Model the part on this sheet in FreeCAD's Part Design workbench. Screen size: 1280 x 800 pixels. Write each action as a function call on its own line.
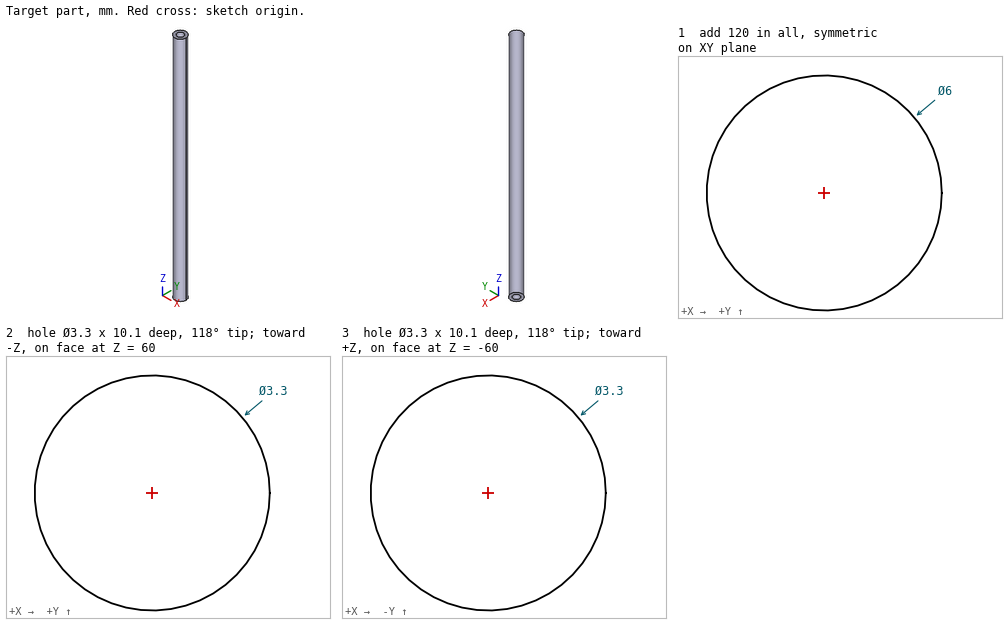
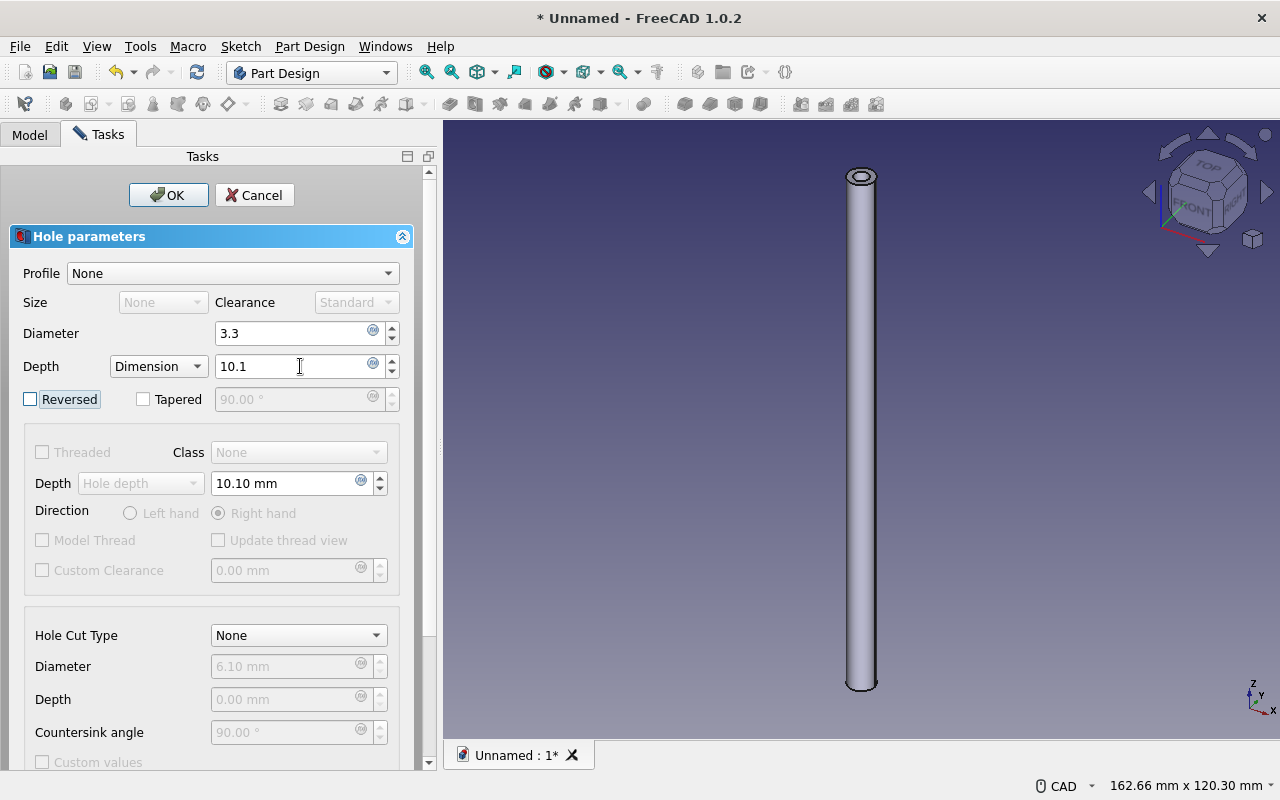
click(169, 195)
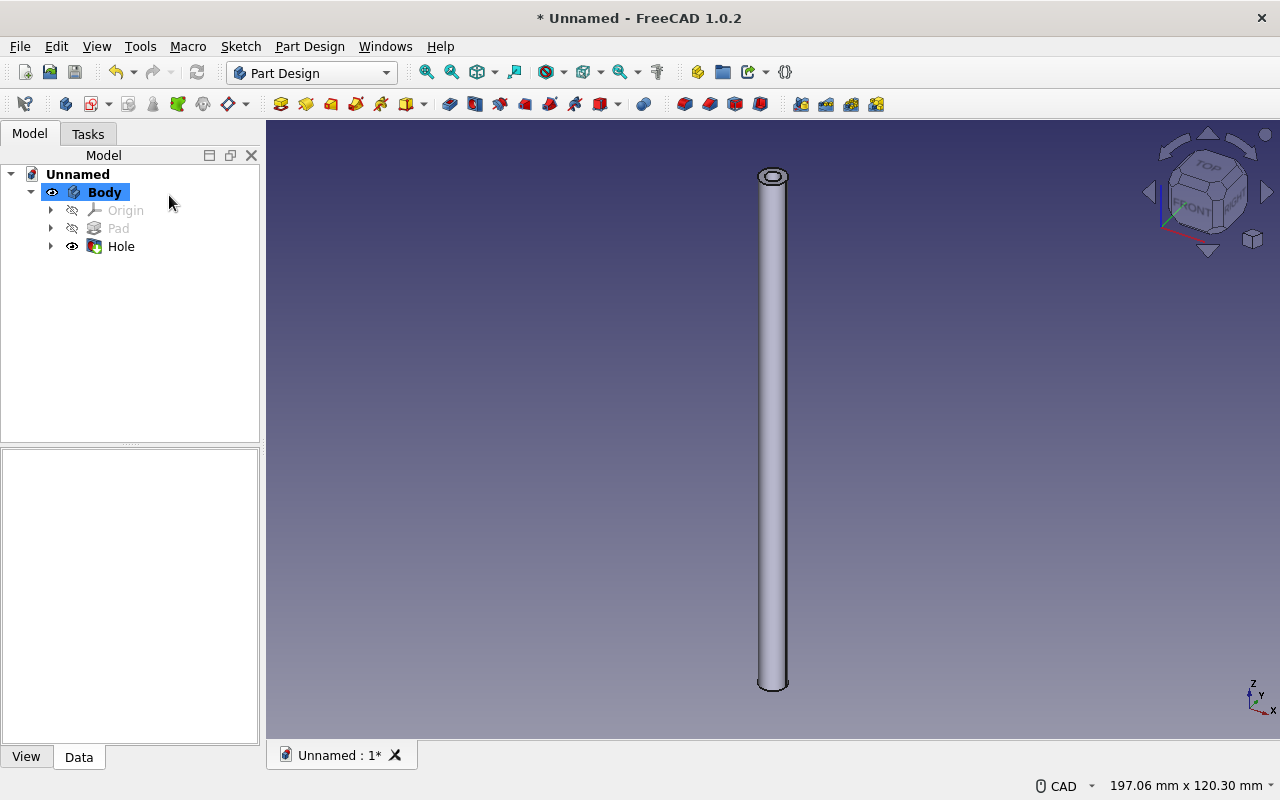
key(5)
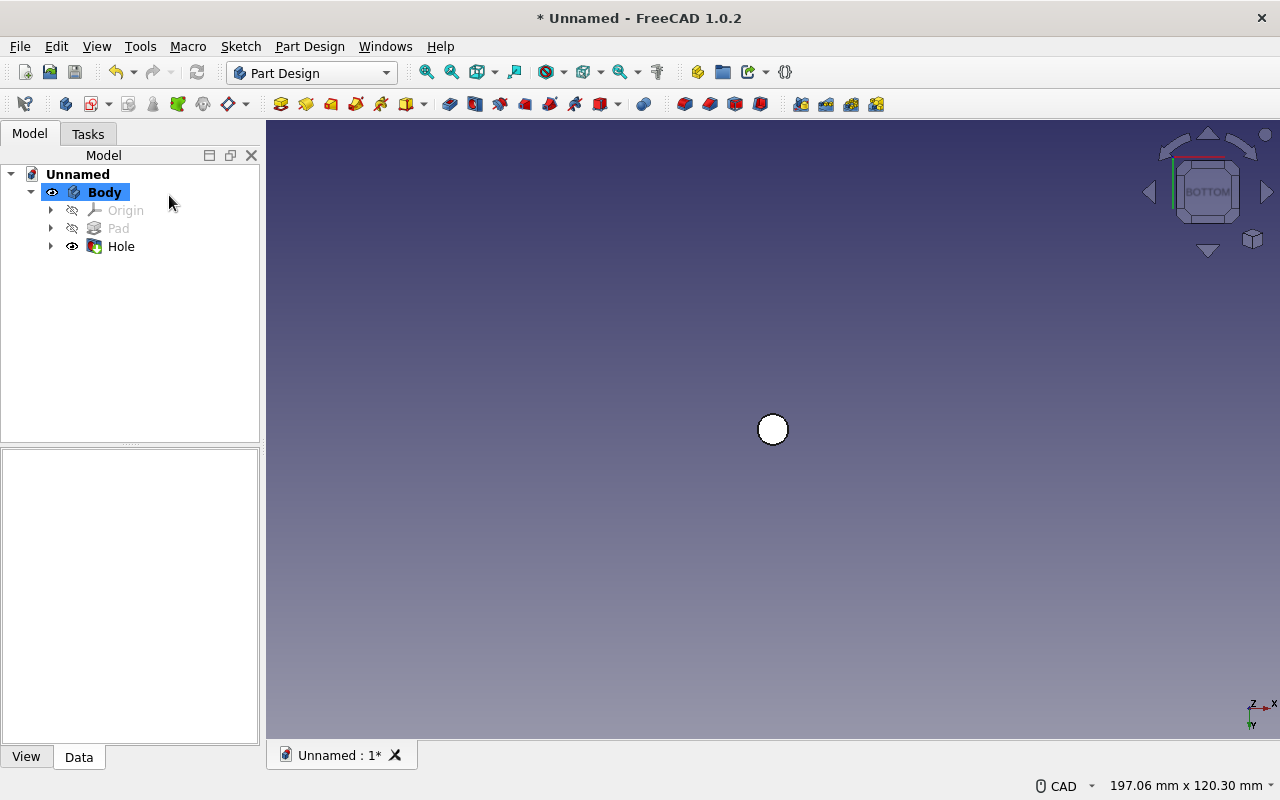
key(v)
key(f)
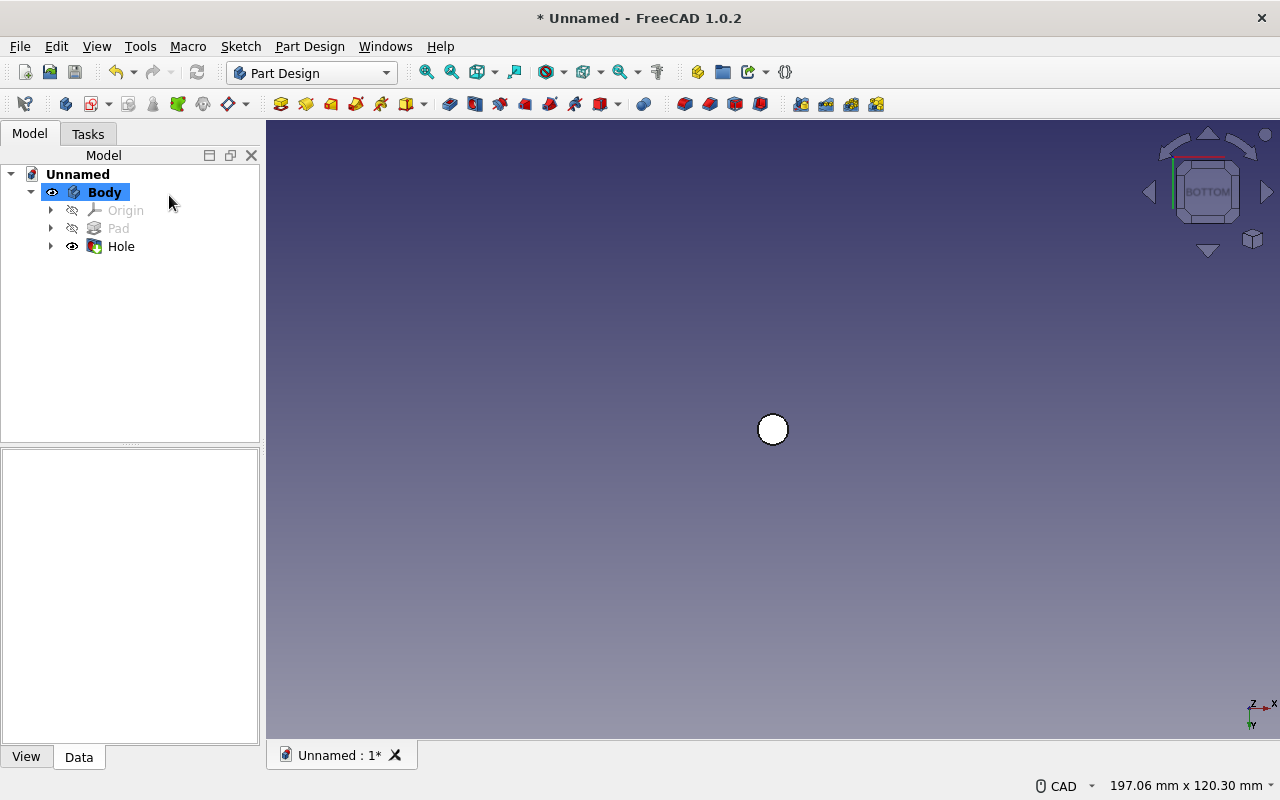
click(773, 428)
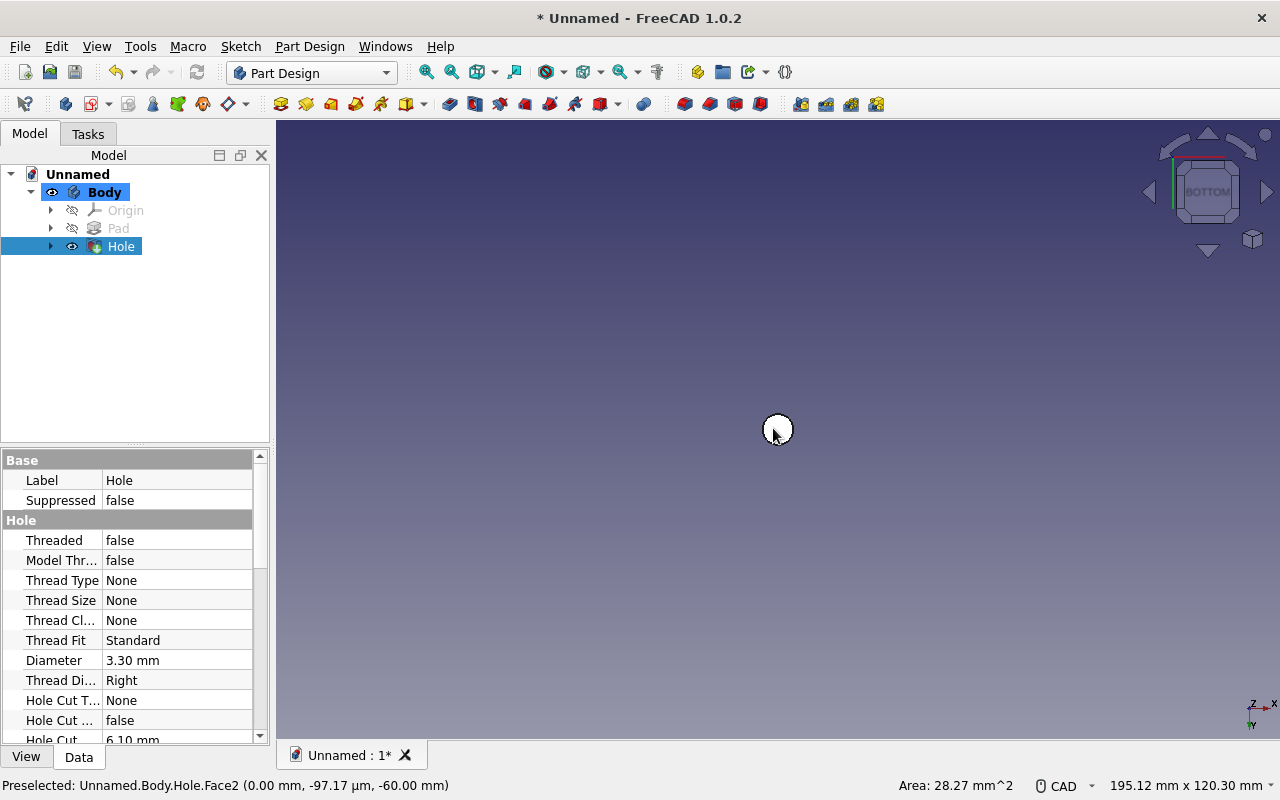
click(90, 104)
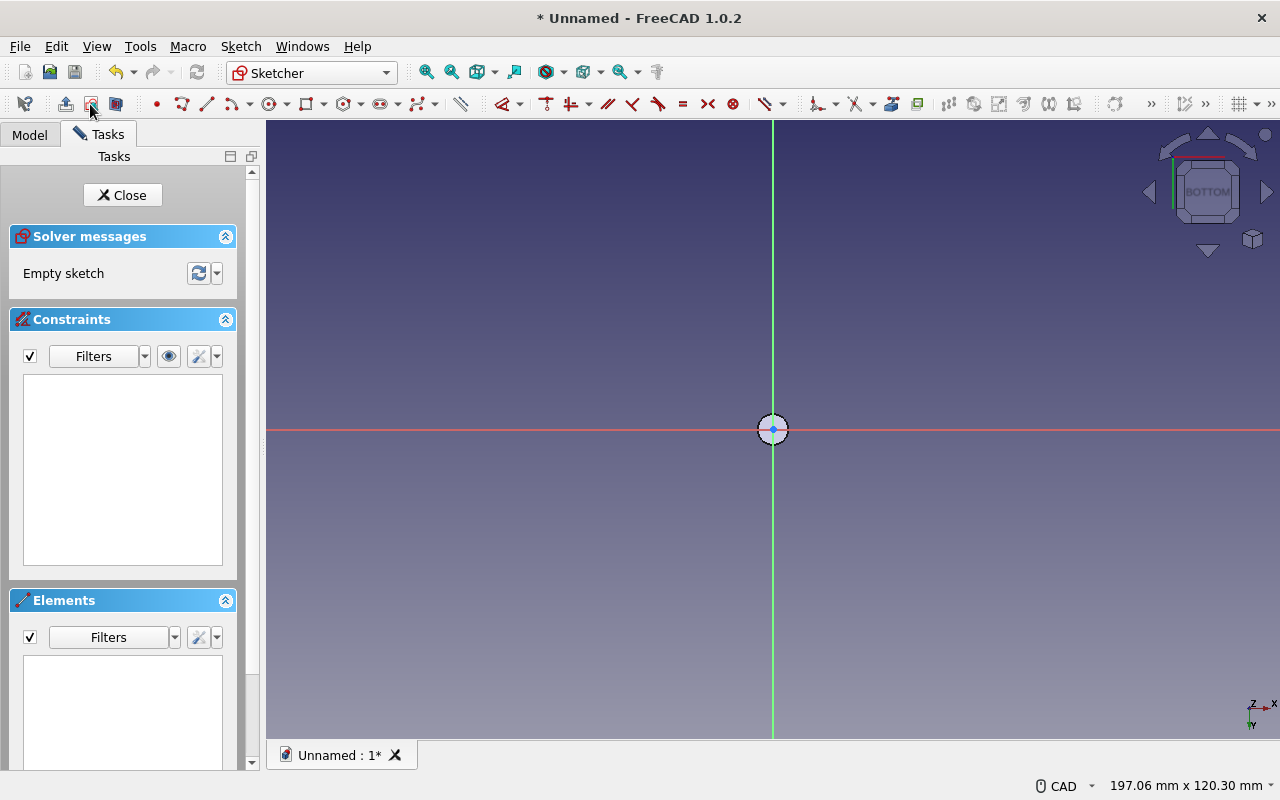
scroll(777, 430, up, 15)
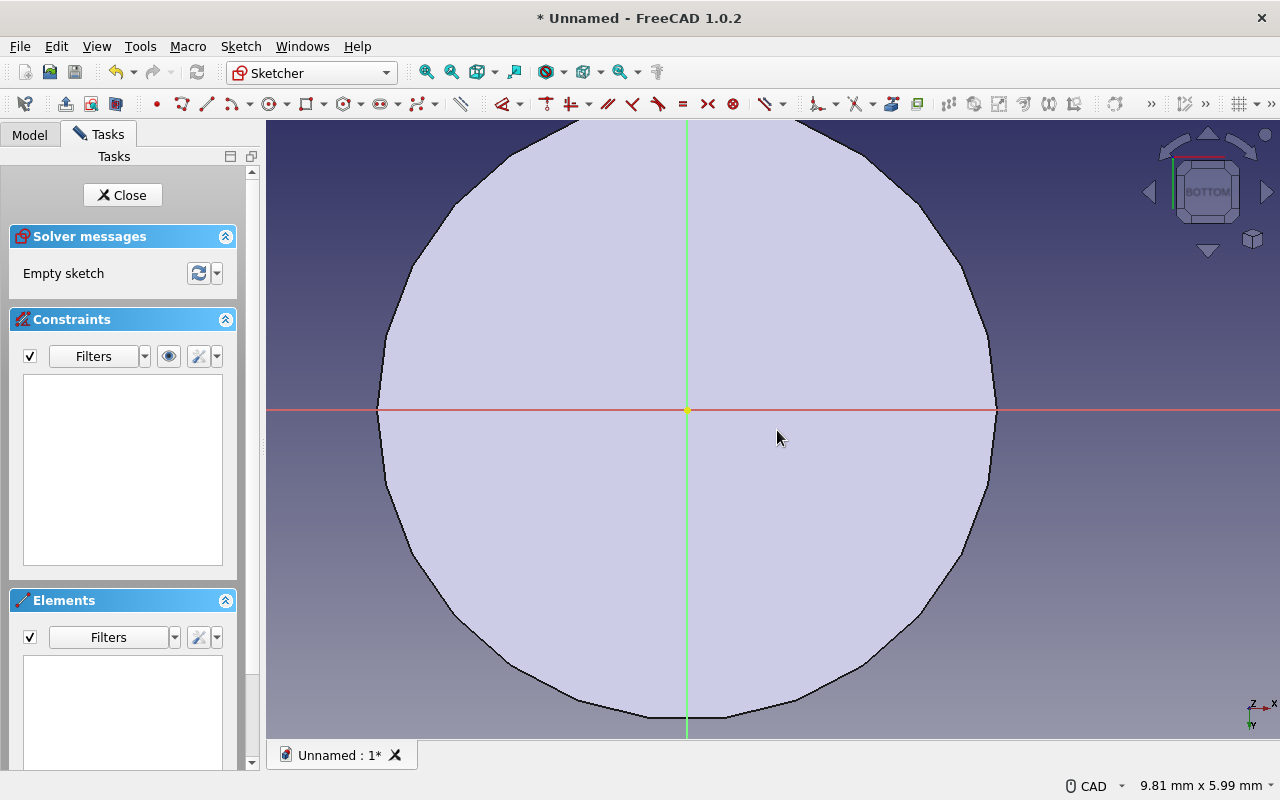
click(268, 104)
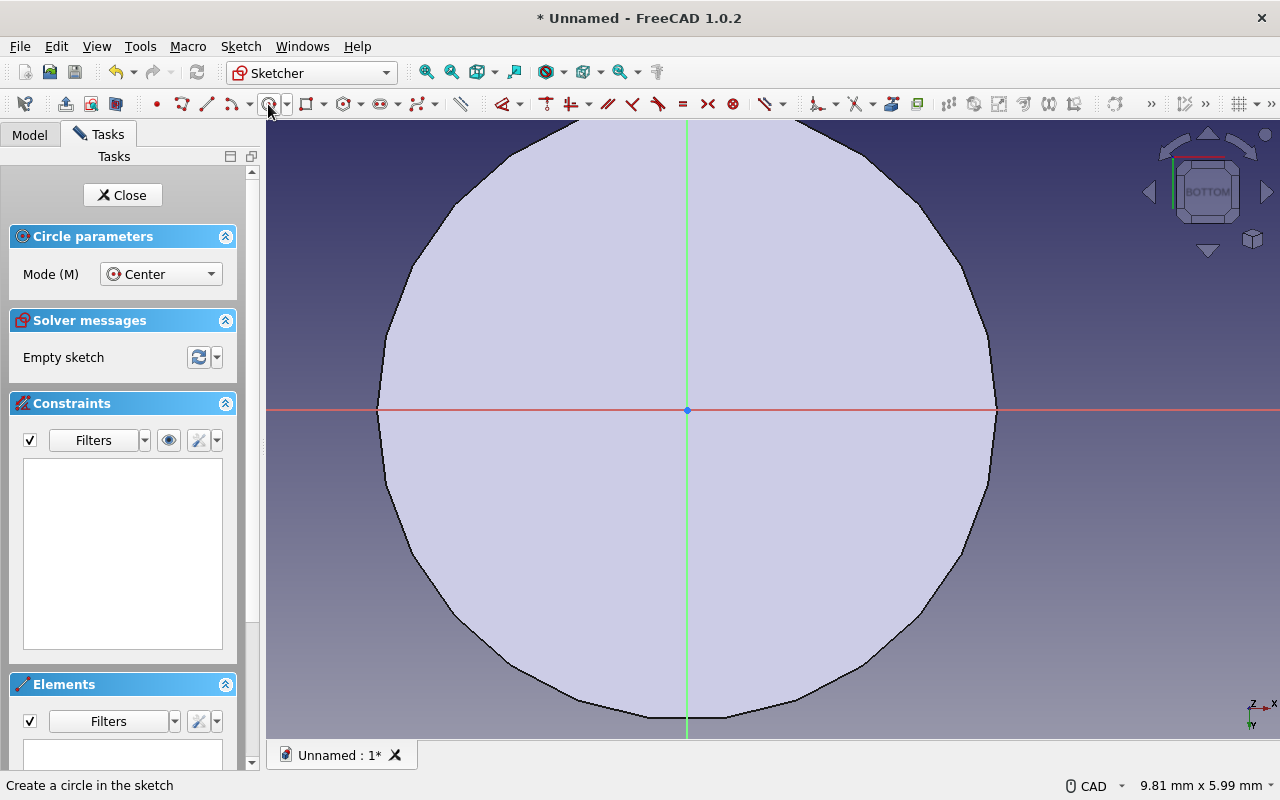
click(687, 410)
click(808, 290)
key(Escape)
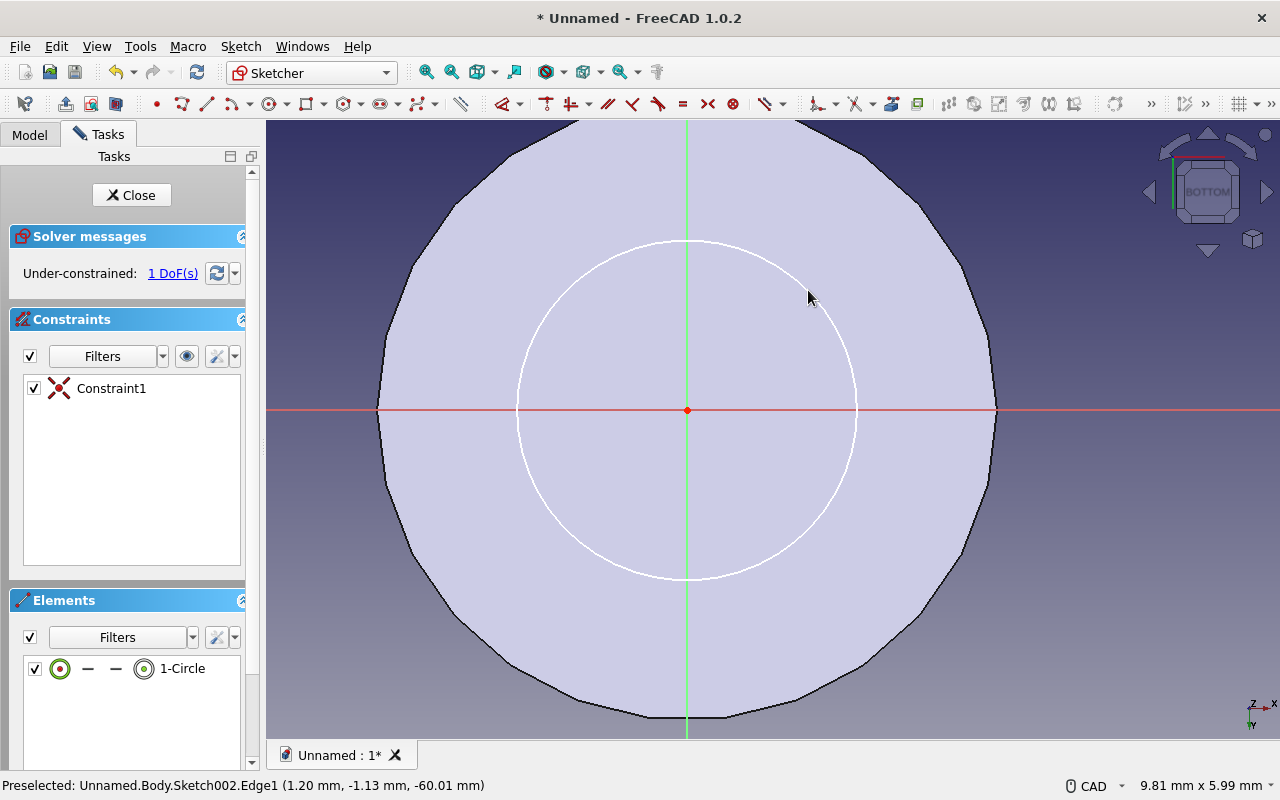
click(502, 104)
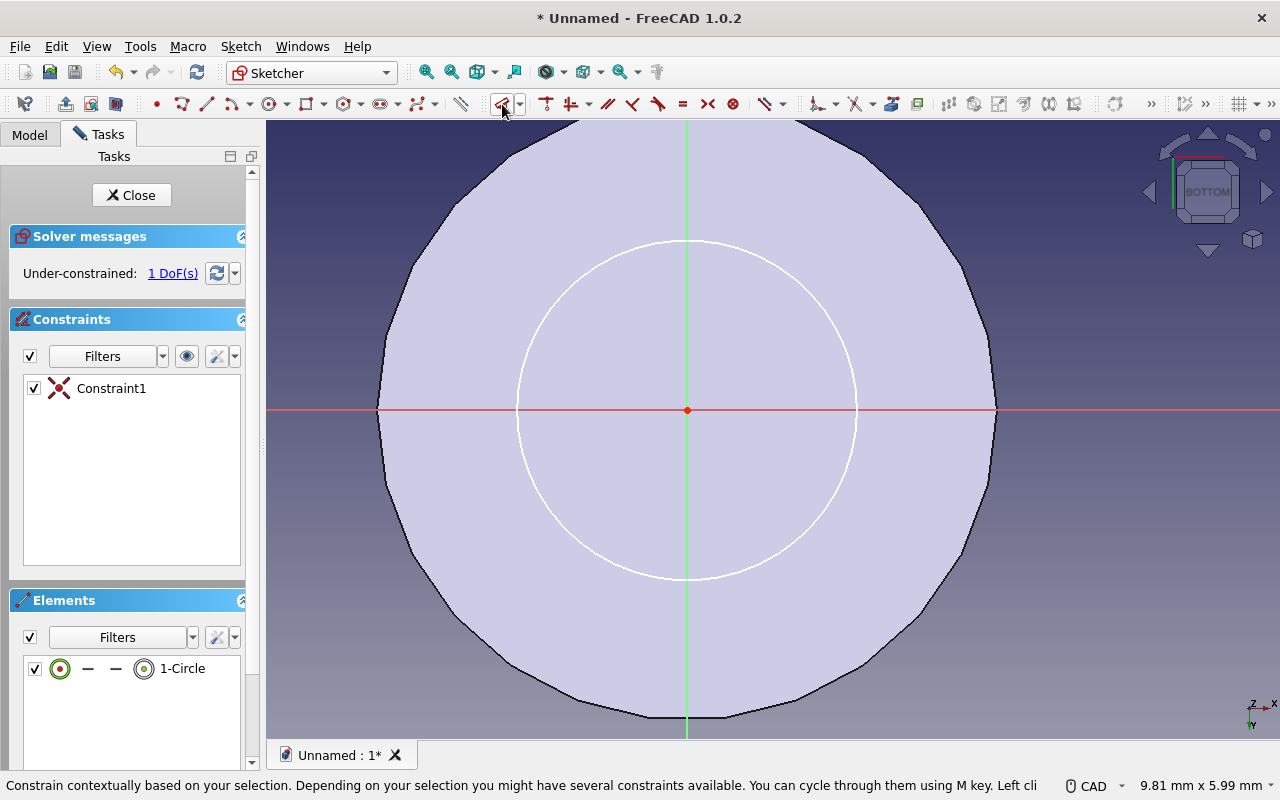
click(807, 290)
click(830, 267)